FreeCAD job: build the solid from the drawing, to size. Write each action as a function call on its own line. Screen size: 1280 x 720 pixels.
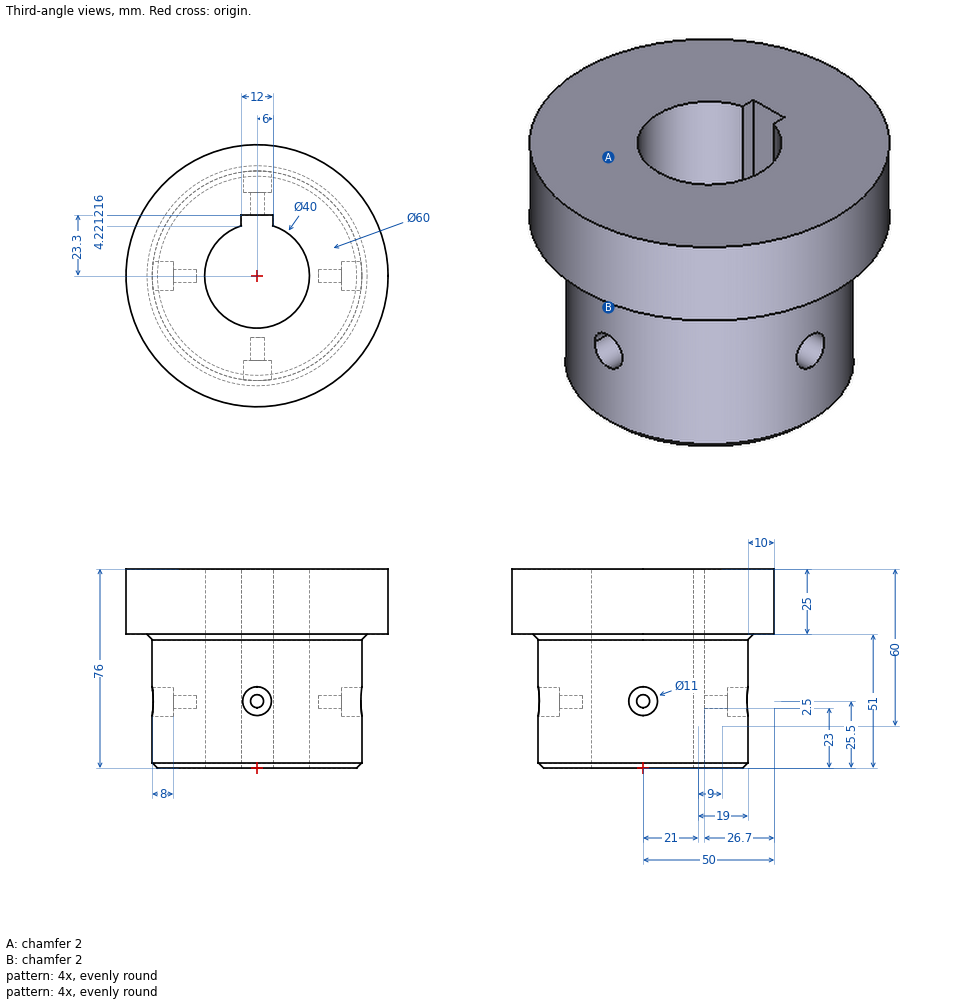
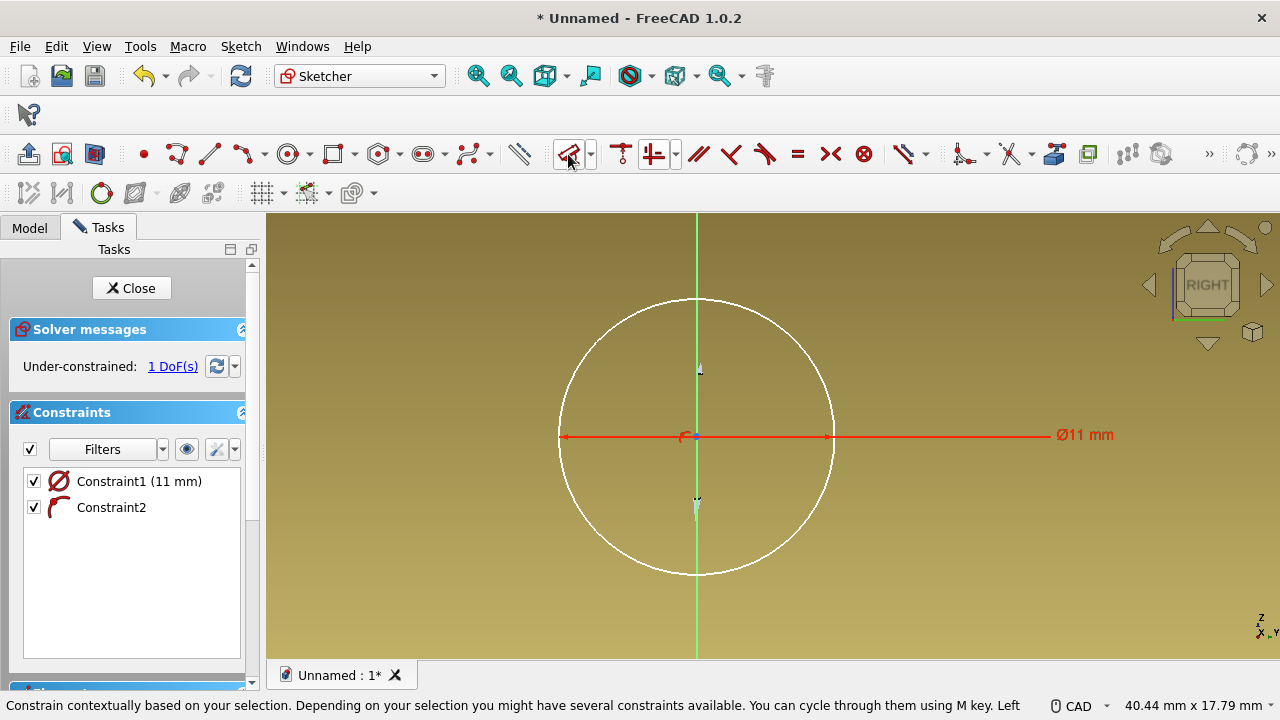
click(697, 437)
click(731, 534)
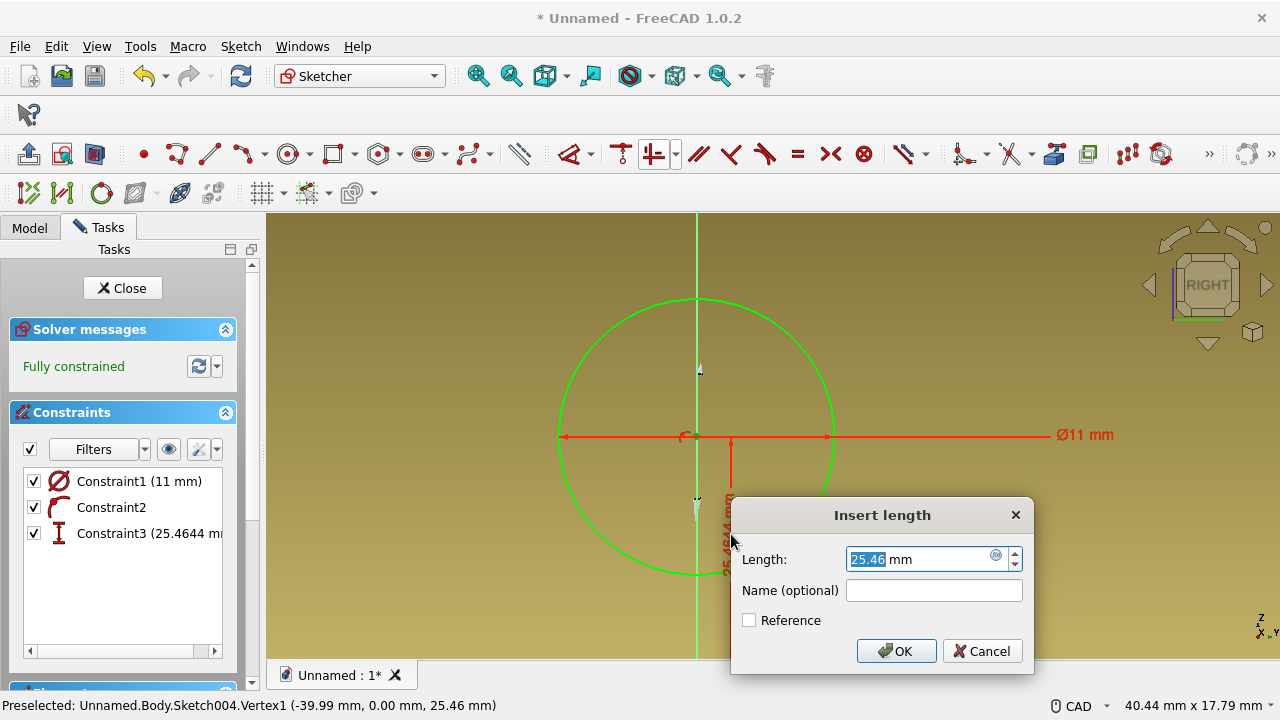
text(25.5)
key(Return)
key(Escape)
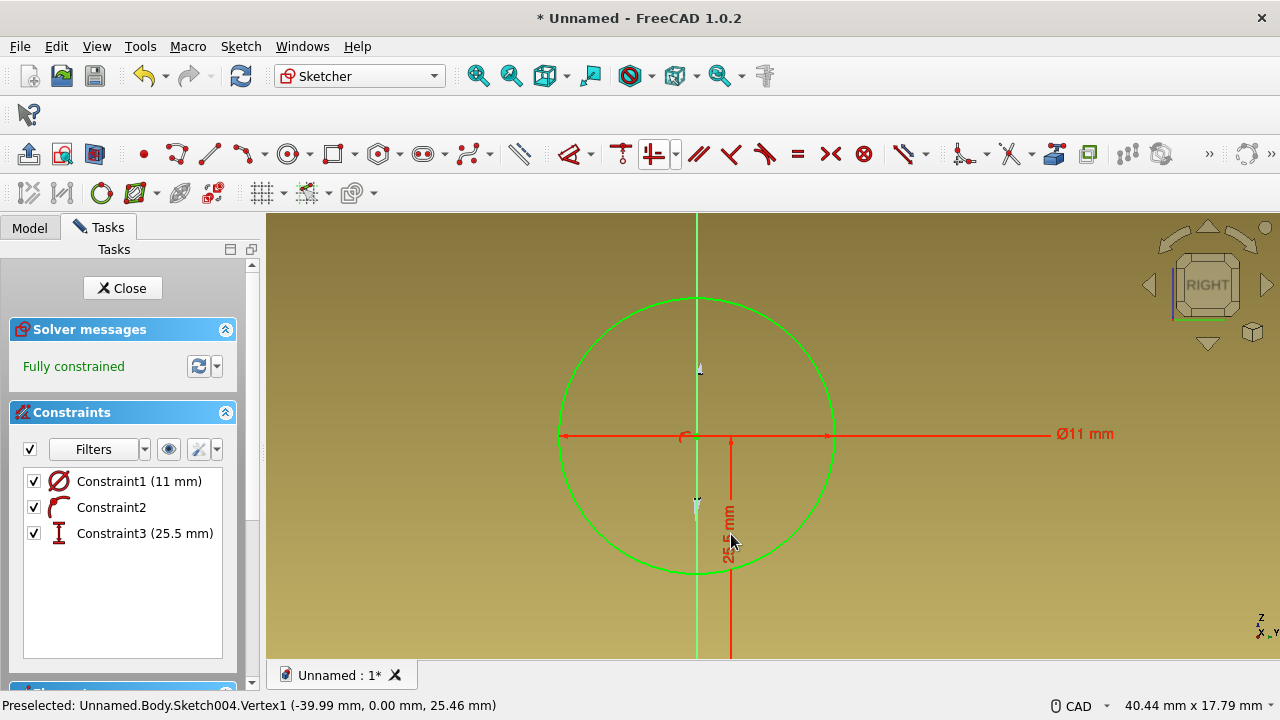
click(123, 288)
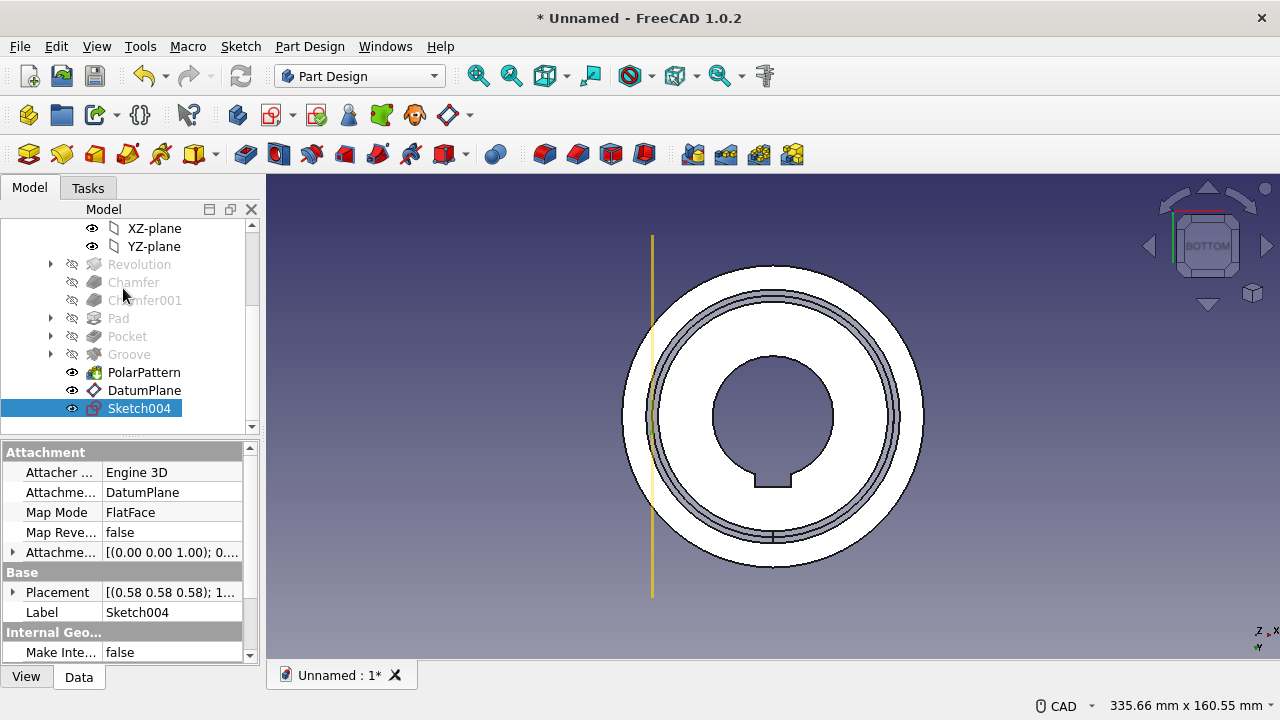
click(246, 154)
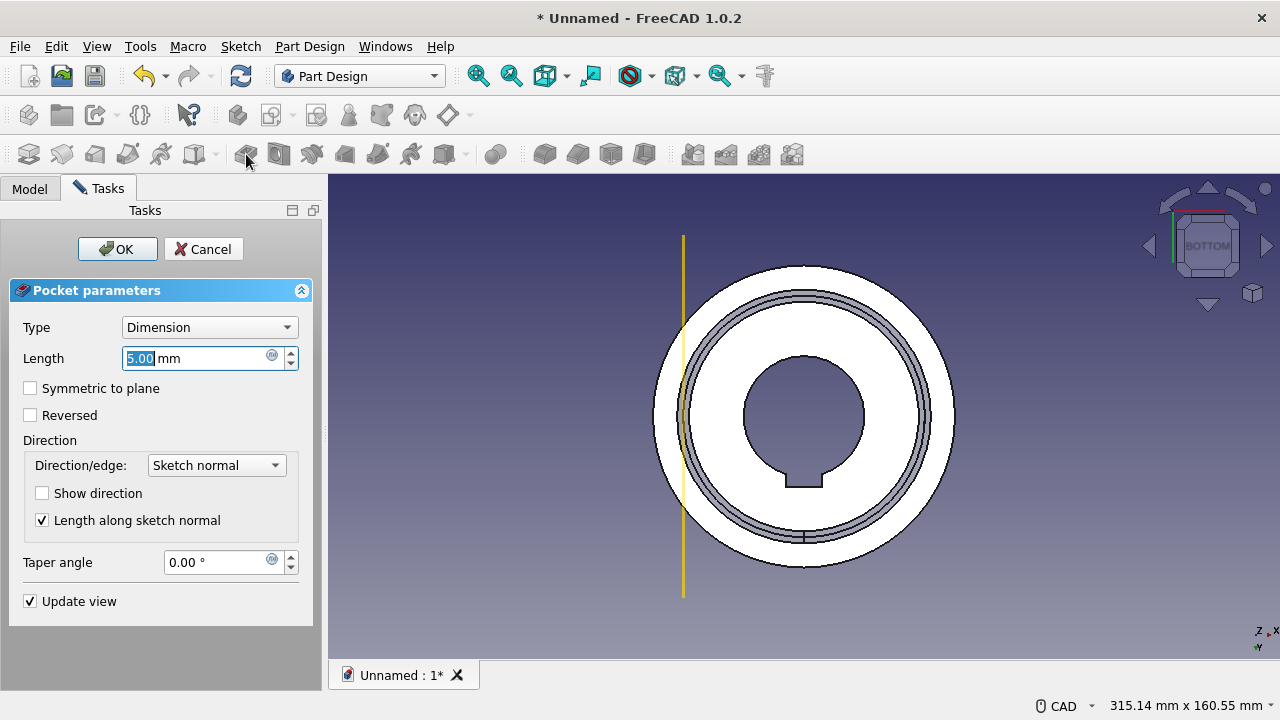
text(8)
key(Tab)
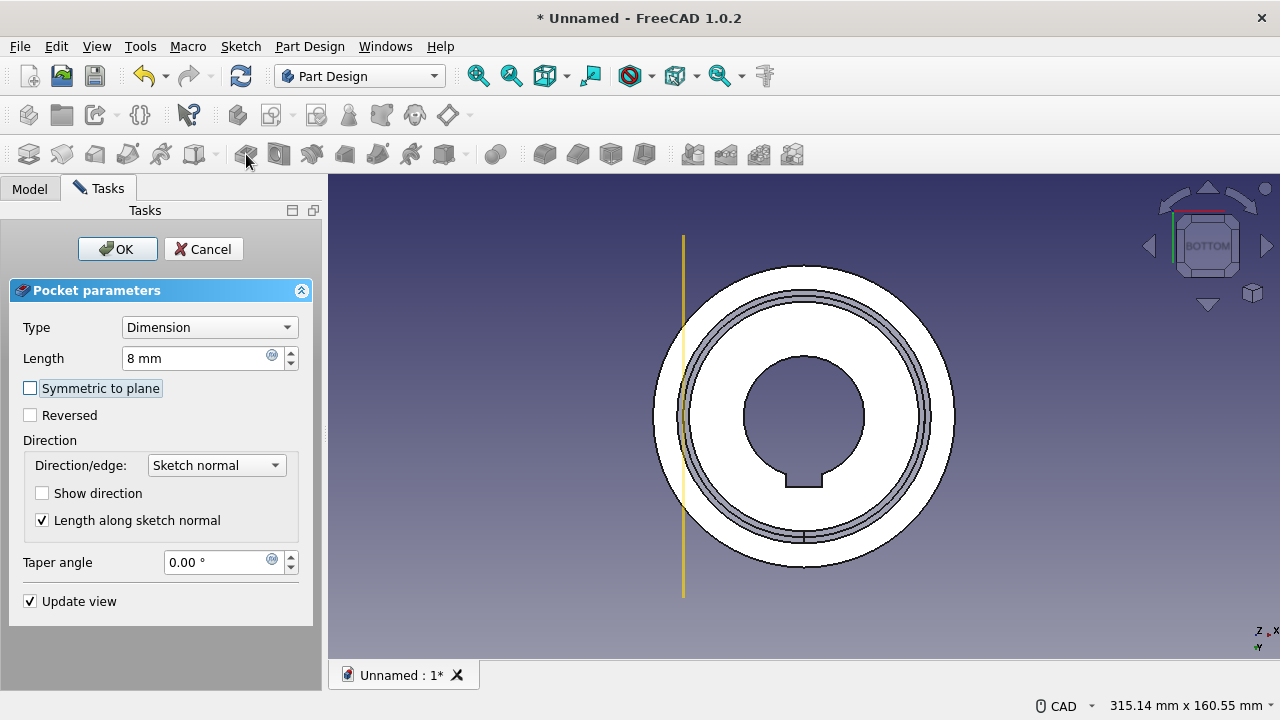
click(31, 415)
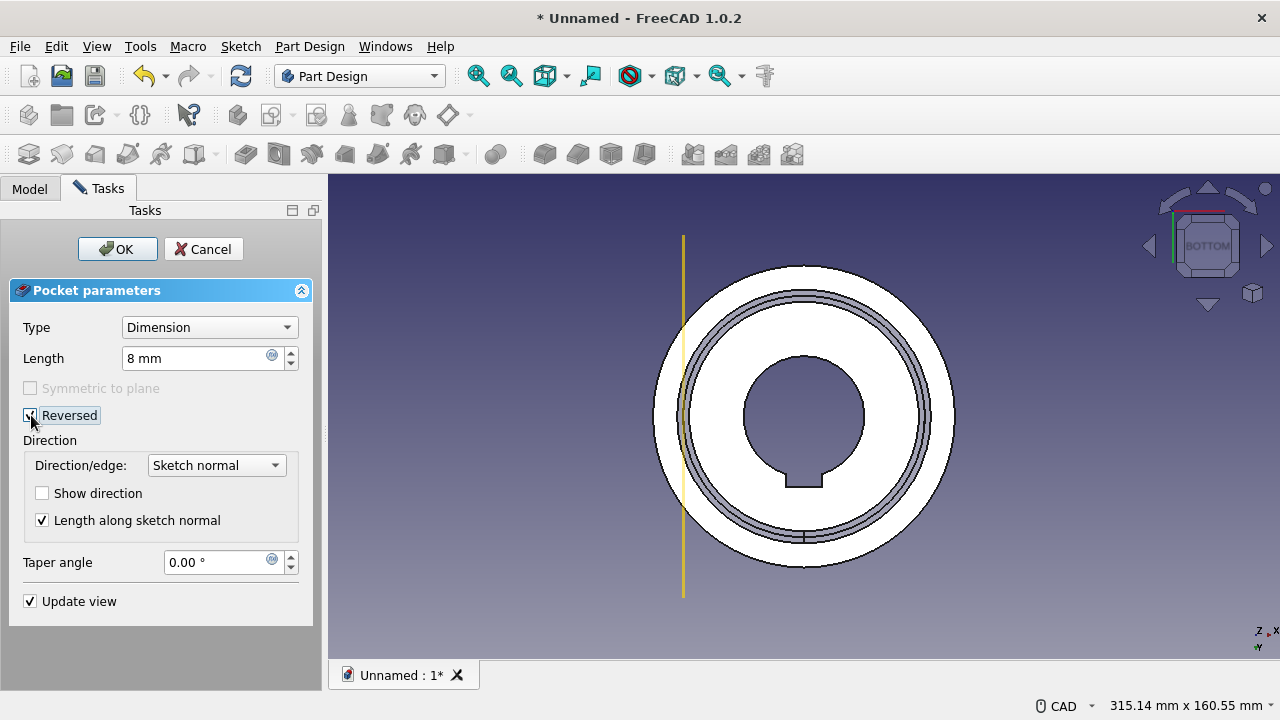
click(118, 249)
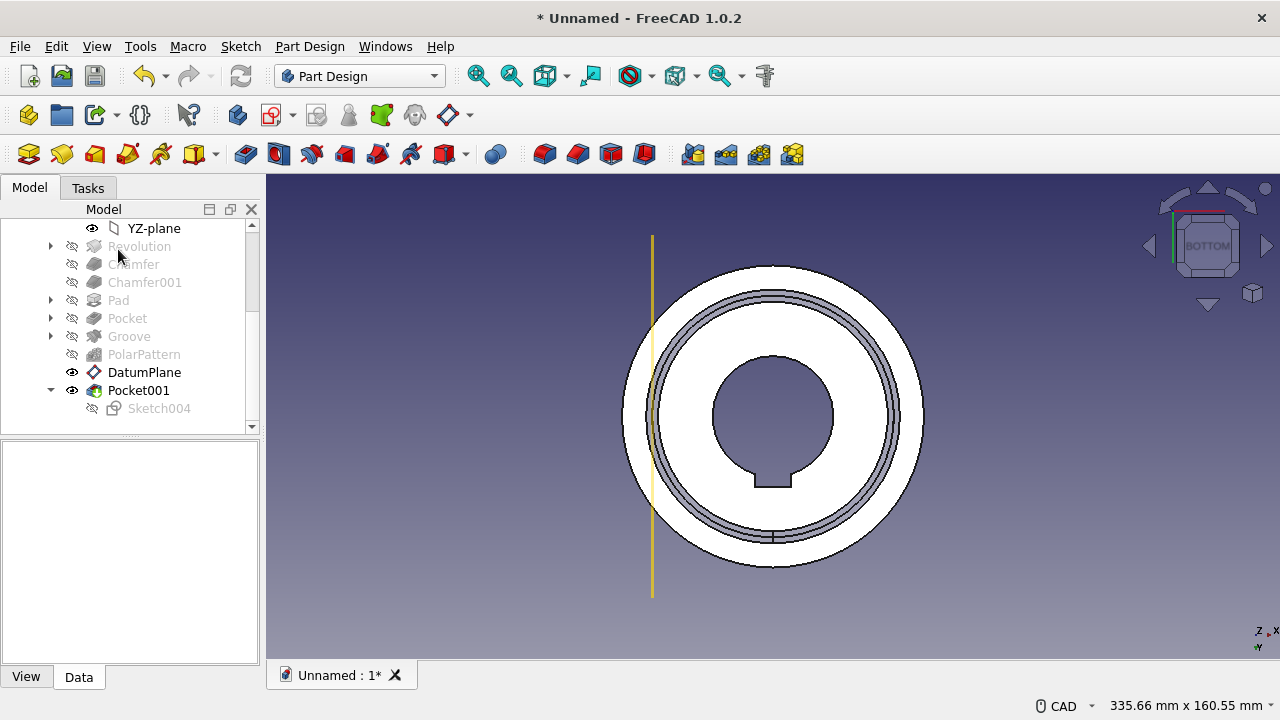
click(117, 372)
key(space)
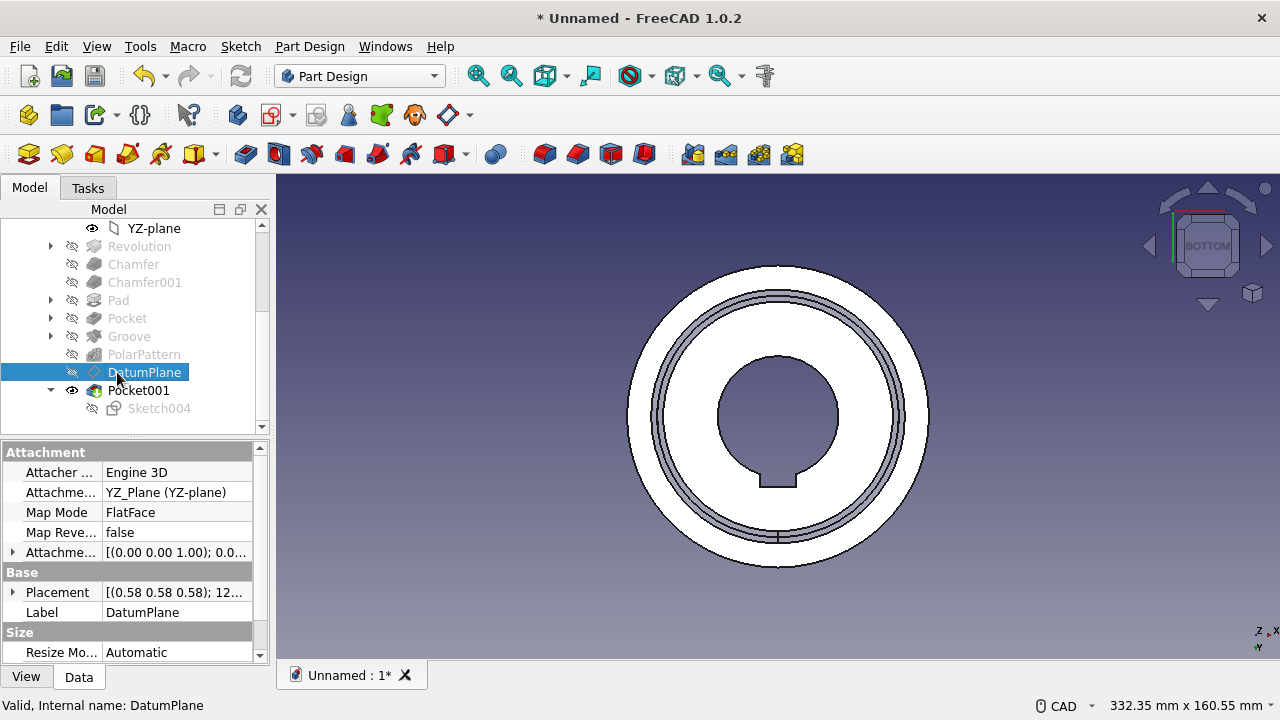
click(117, 390)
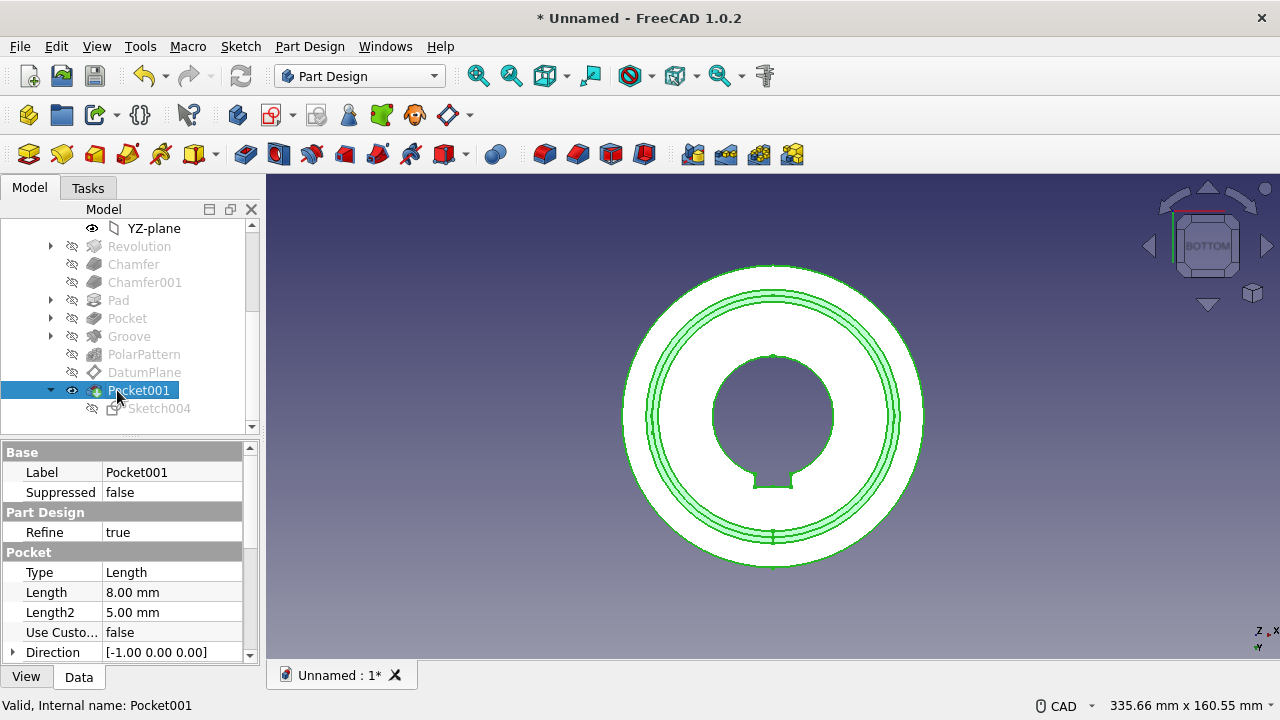
click(759, 154)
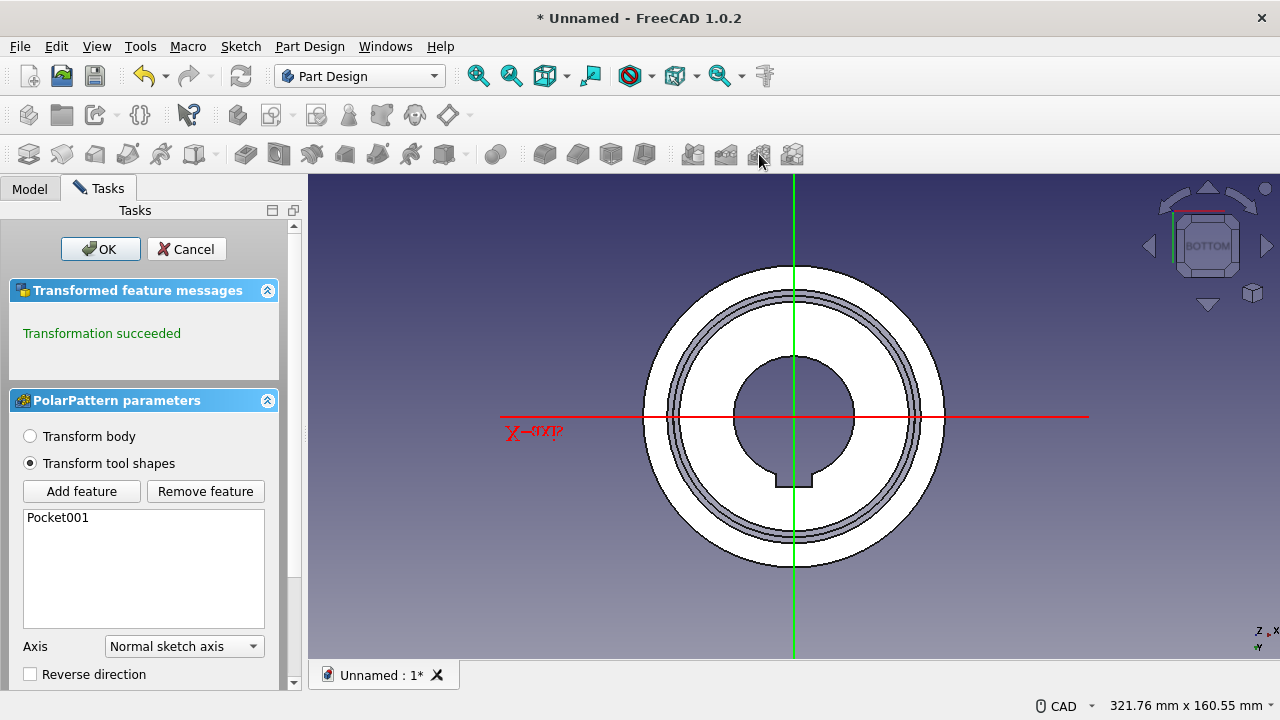
click(185, 646)